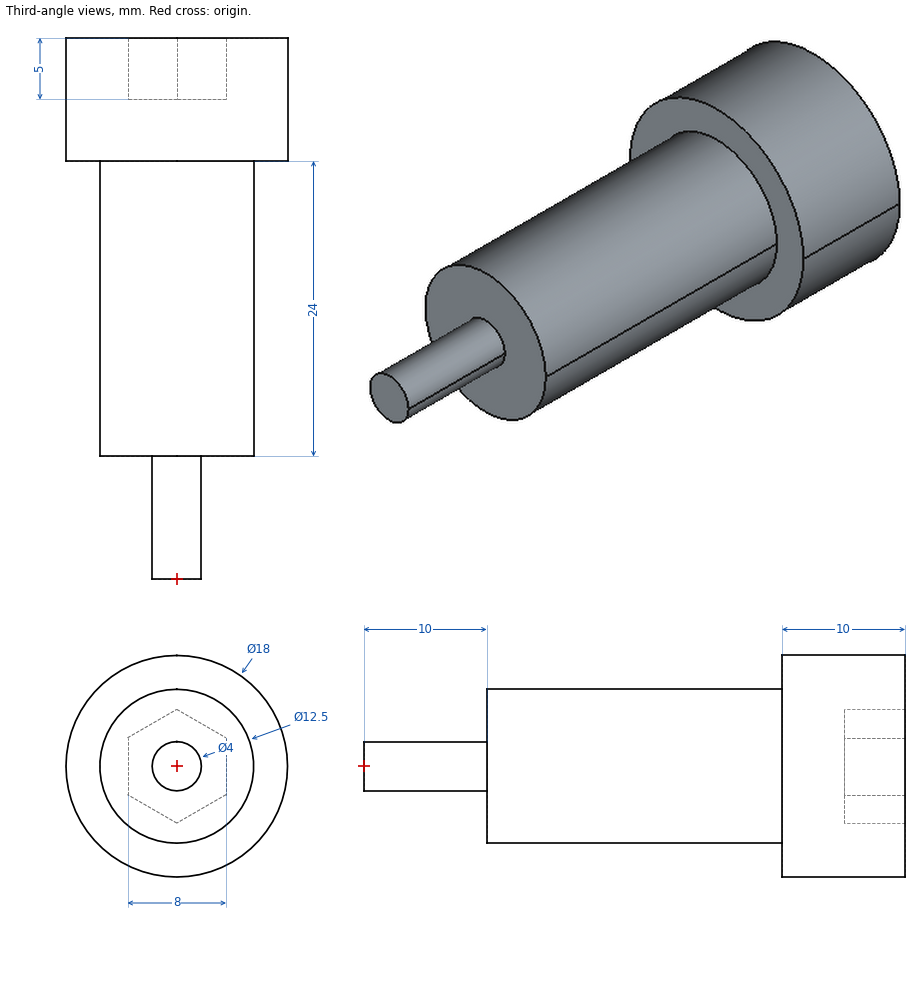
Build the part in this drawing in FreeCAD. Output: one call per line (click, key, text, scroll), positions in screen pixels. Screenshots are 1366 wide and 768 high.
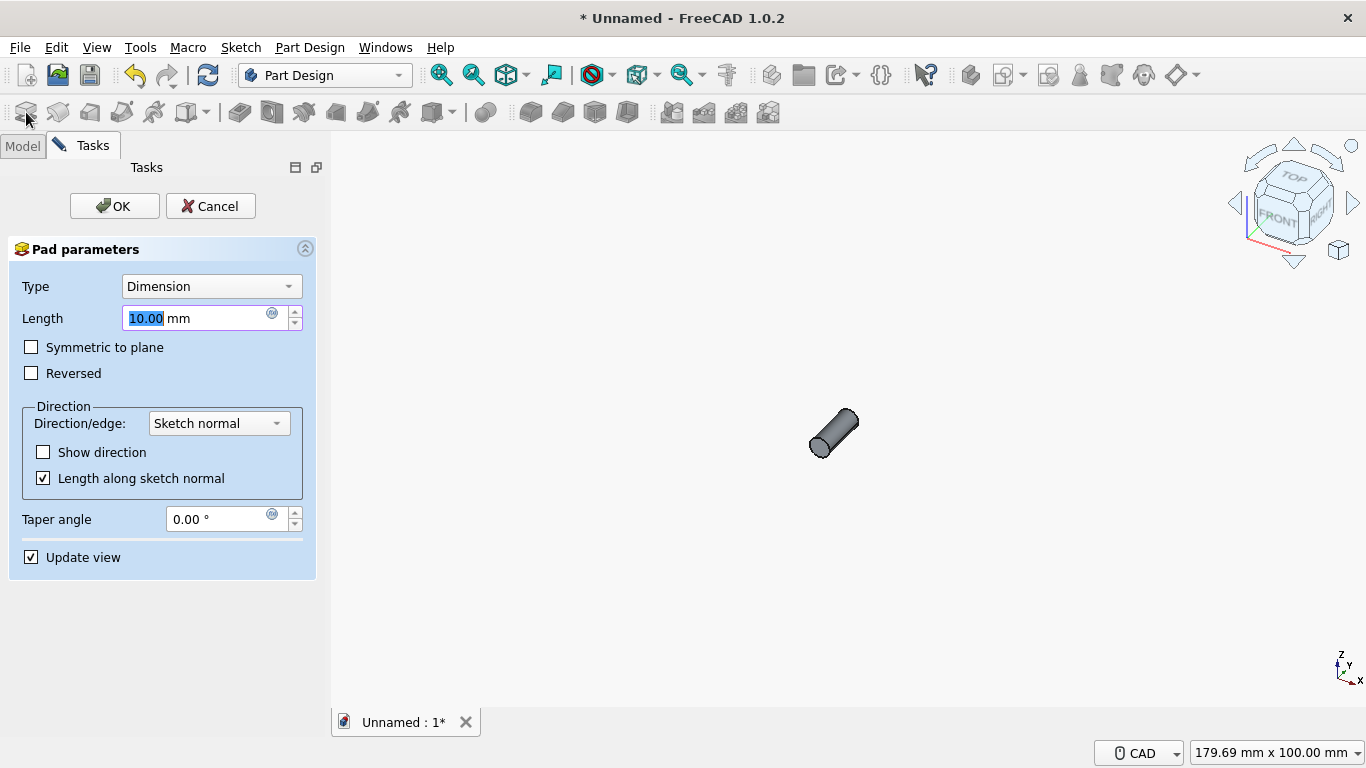
text(10)
key(Tab)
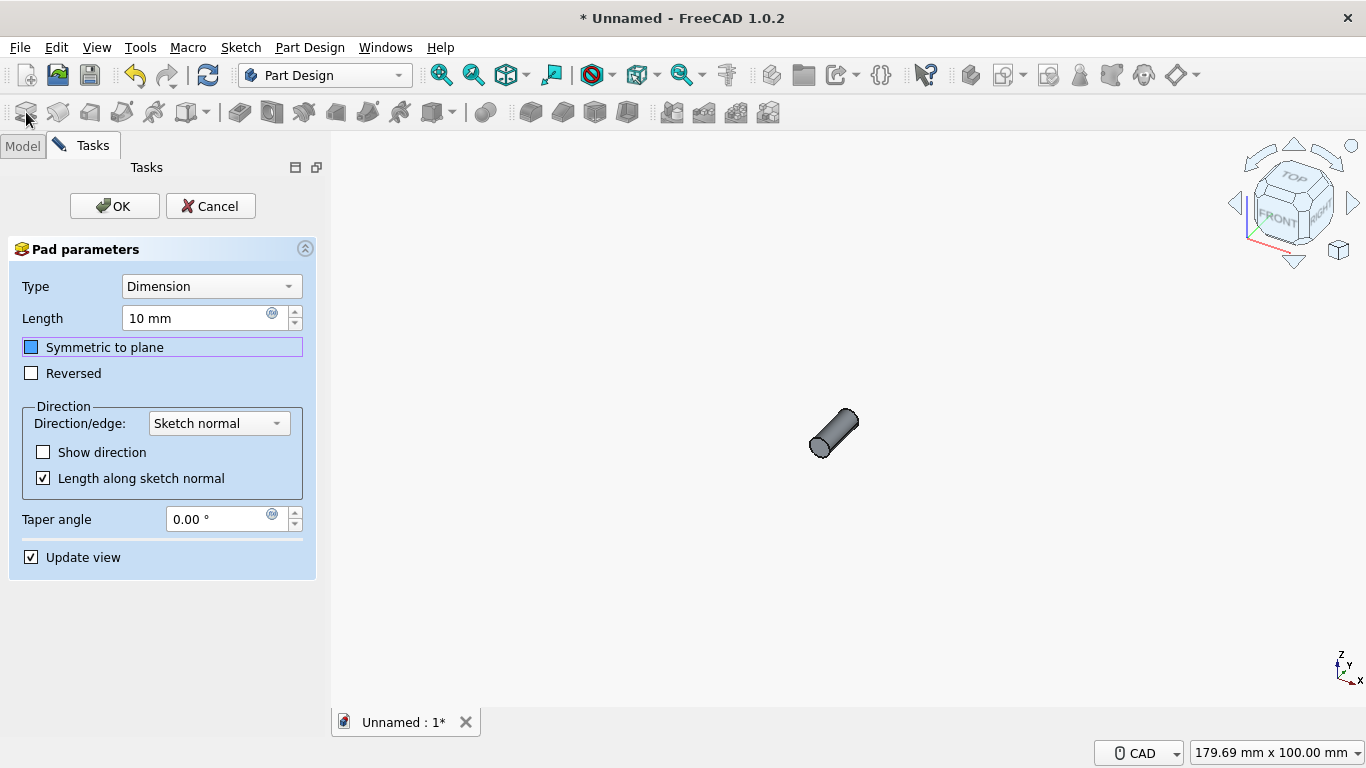
click(30, 373)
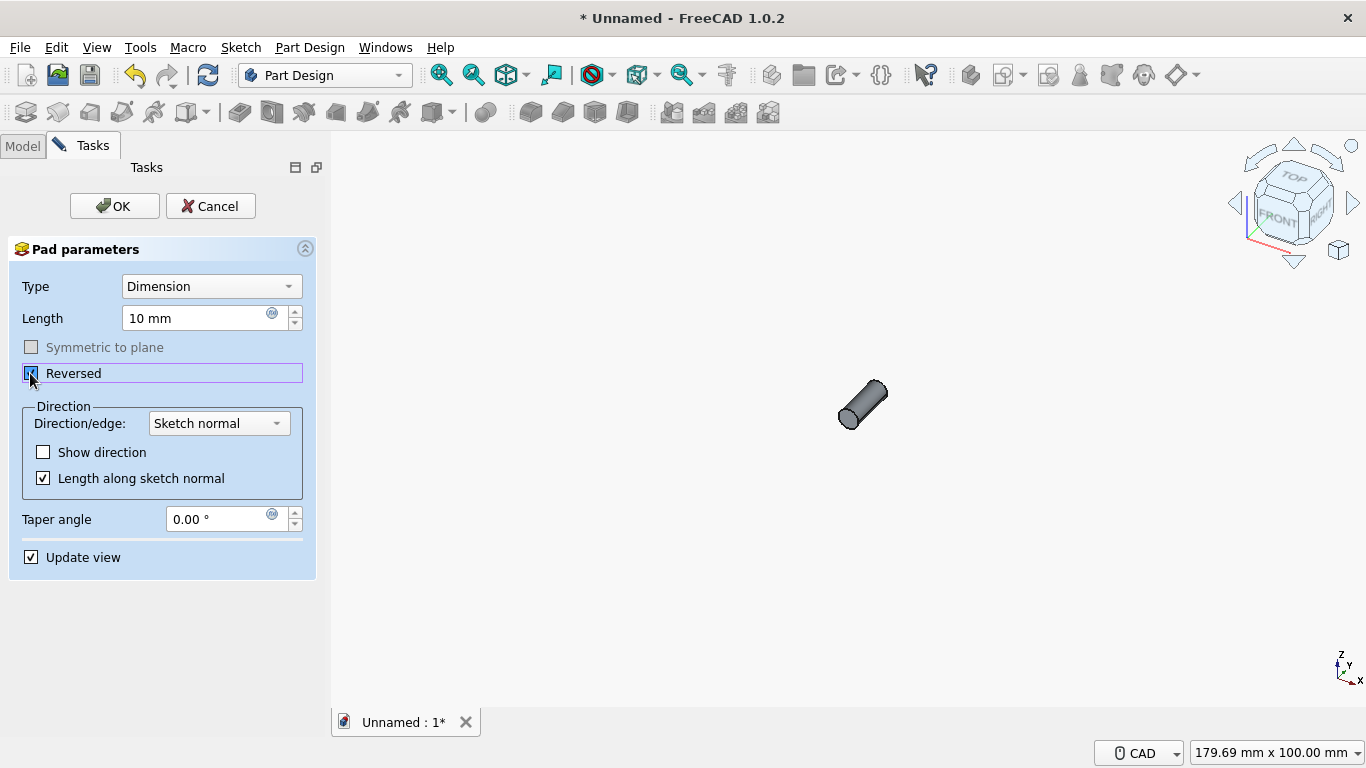
click(115, 206)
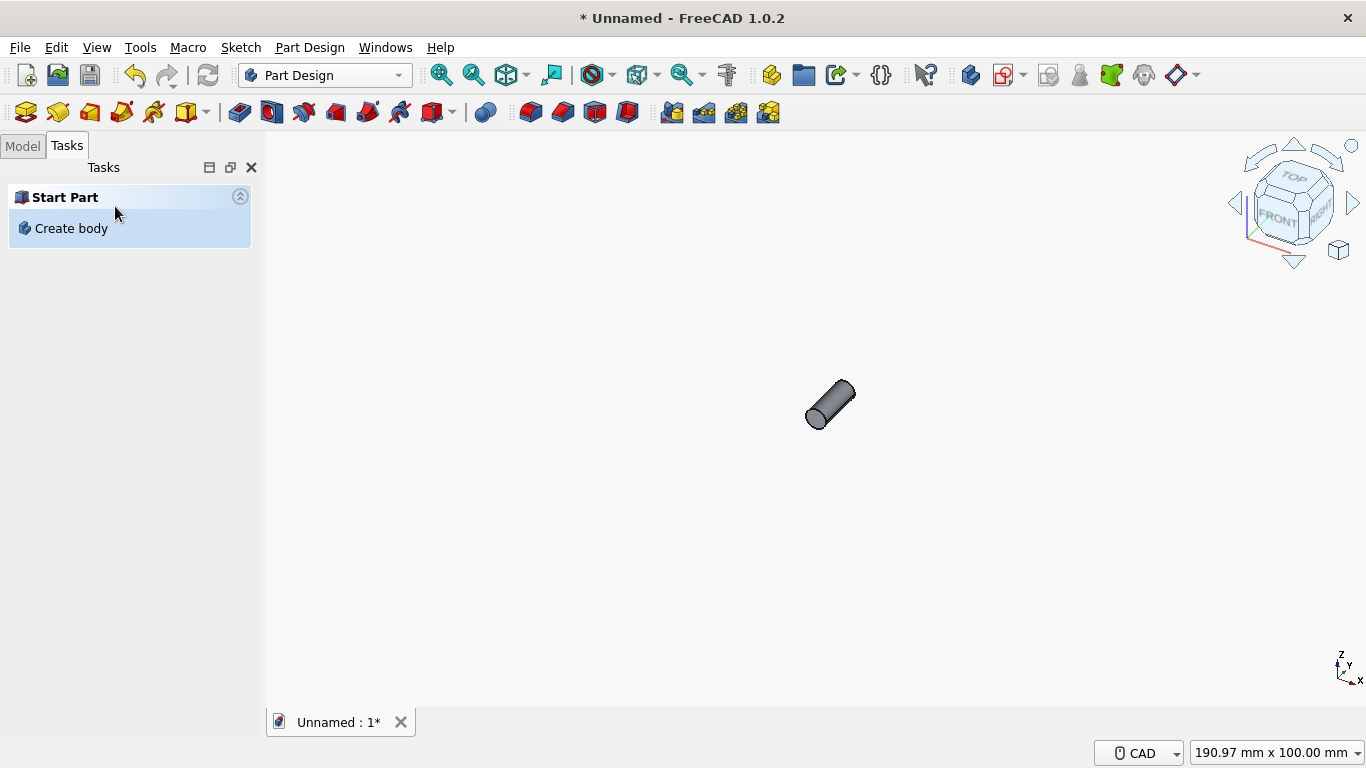
key(v)
key(f)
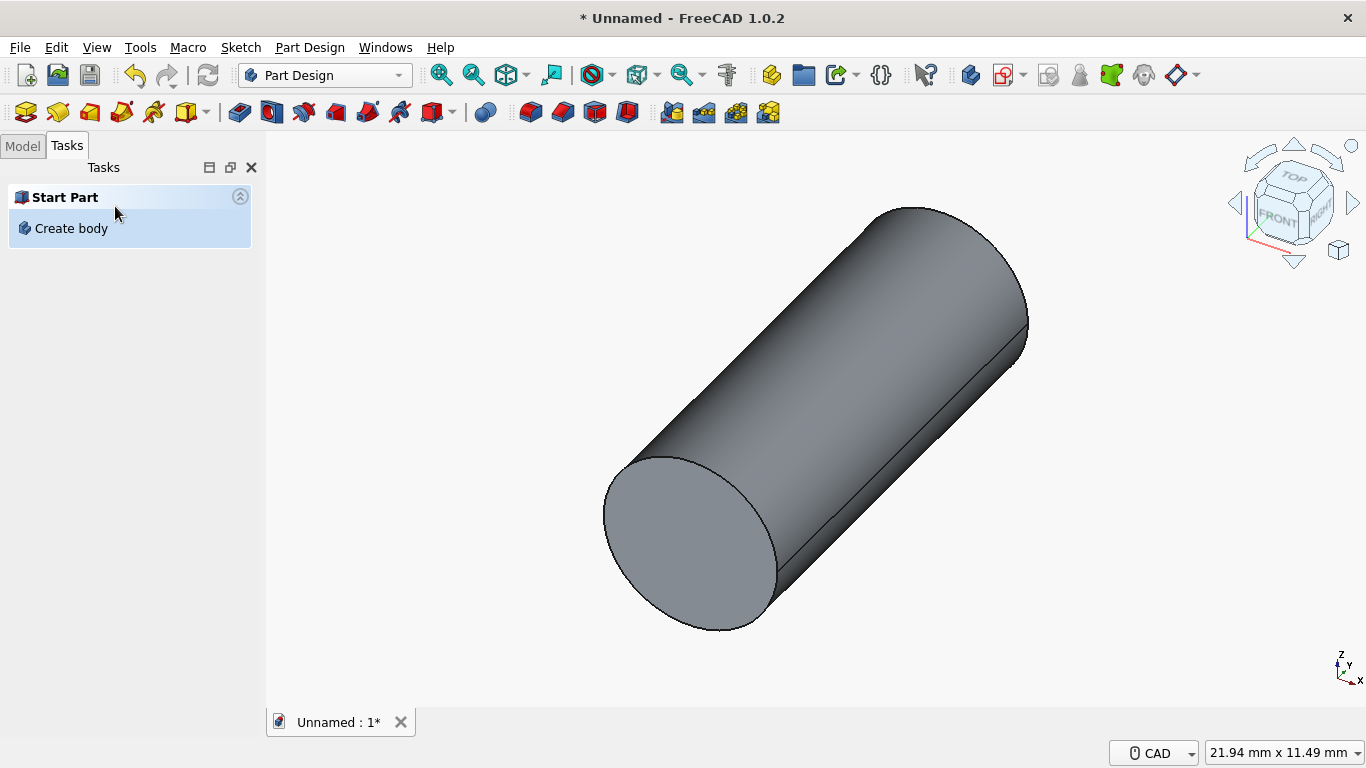
key(4)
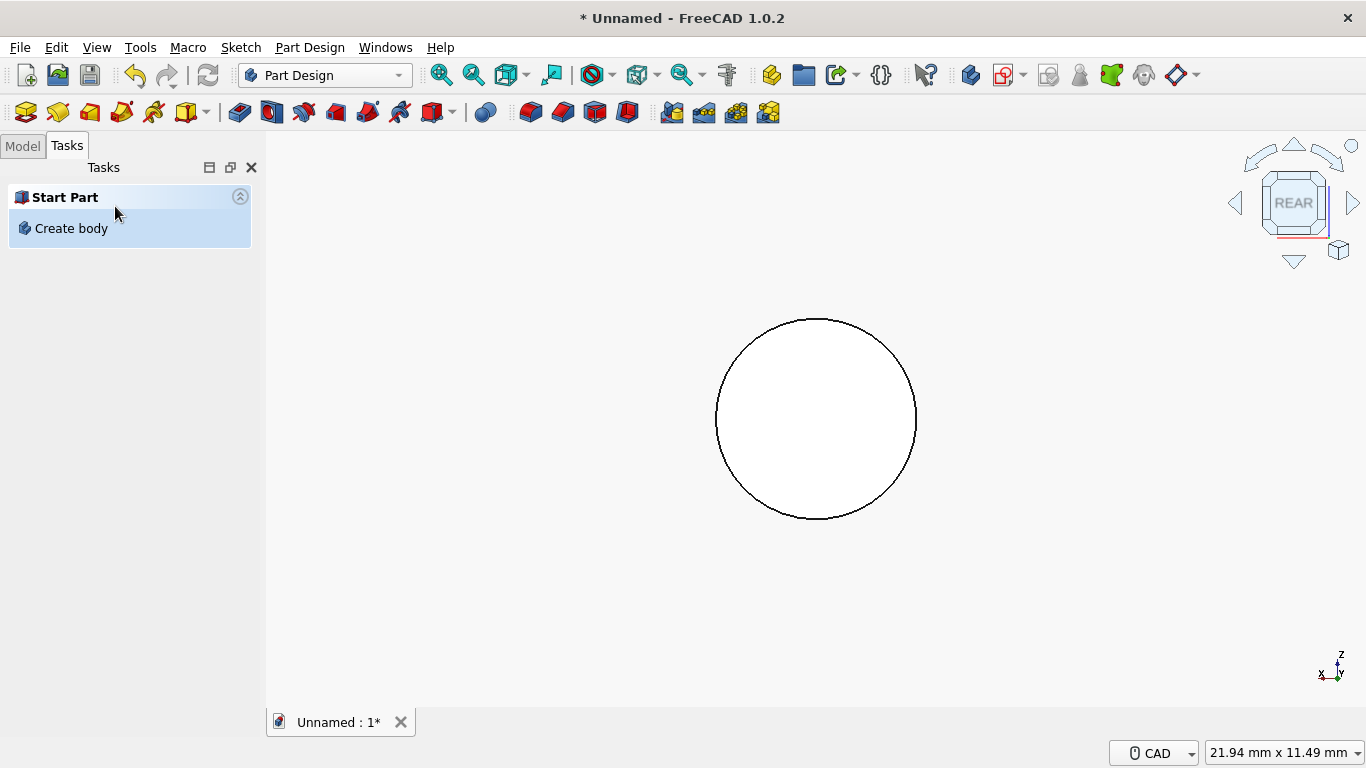
key(v)
key(f)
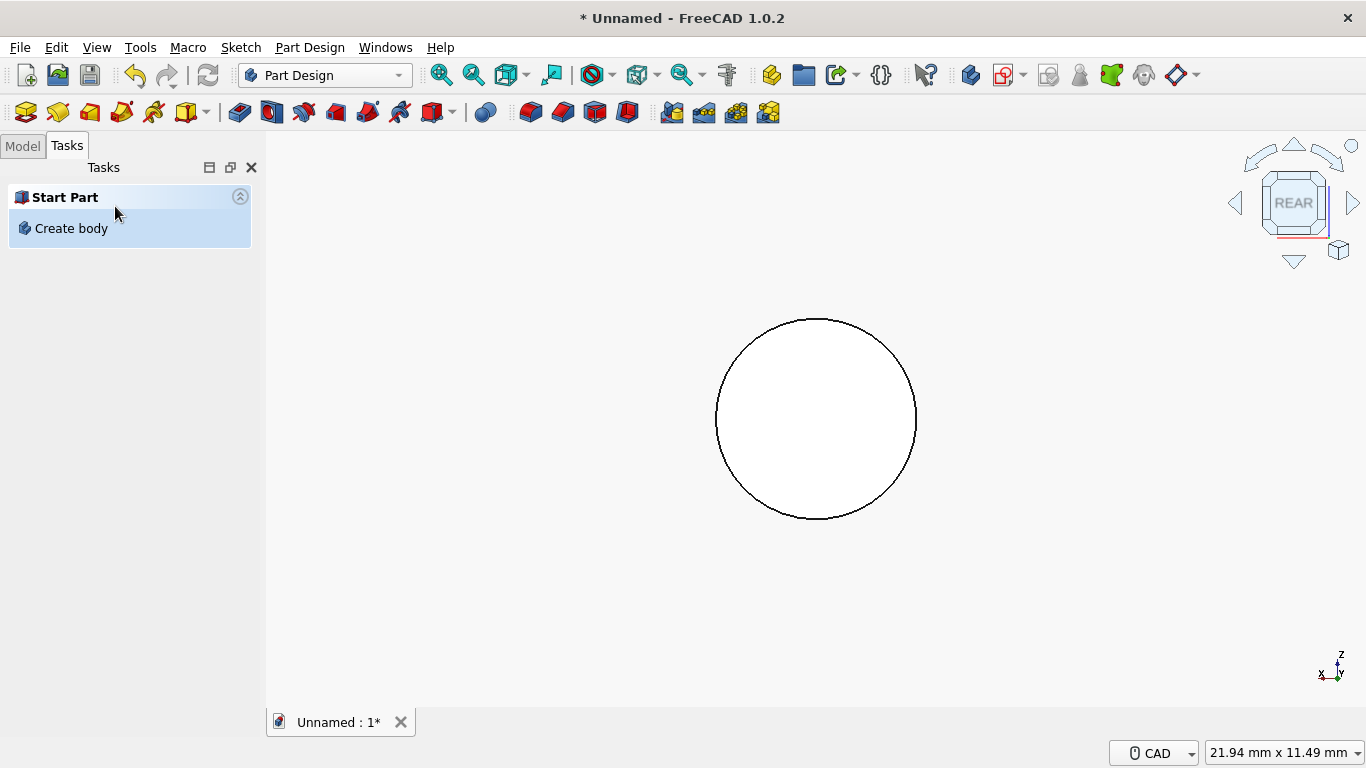
click(816, 418)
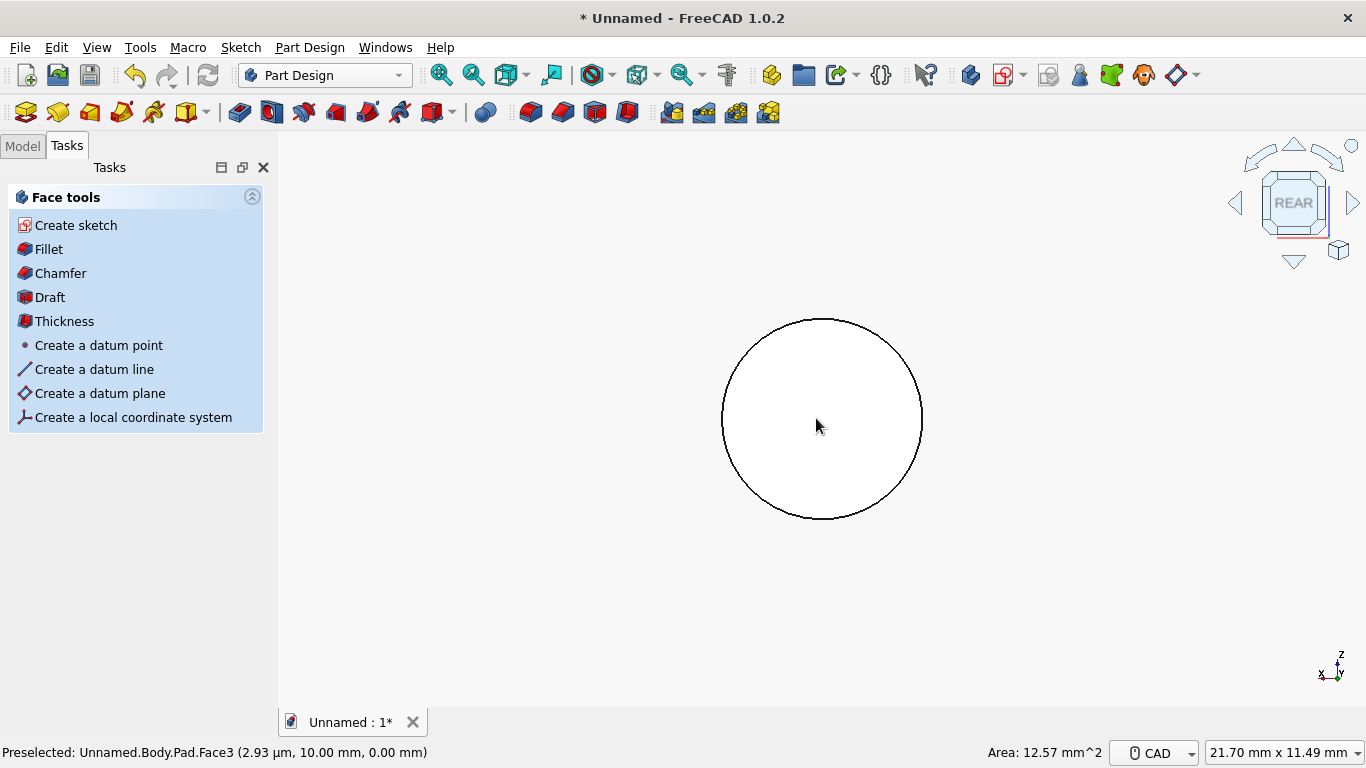
click(1004, 76)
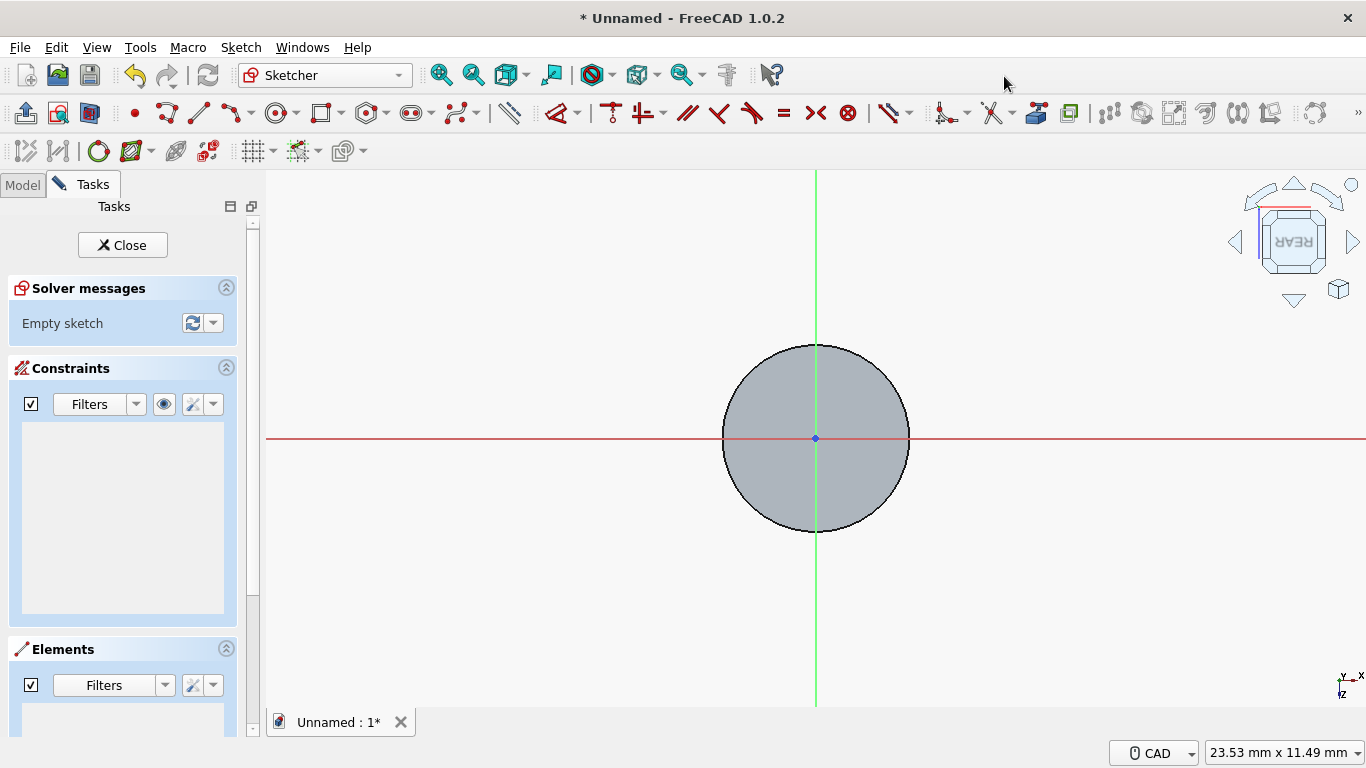
scroll(664, 439, down, 3)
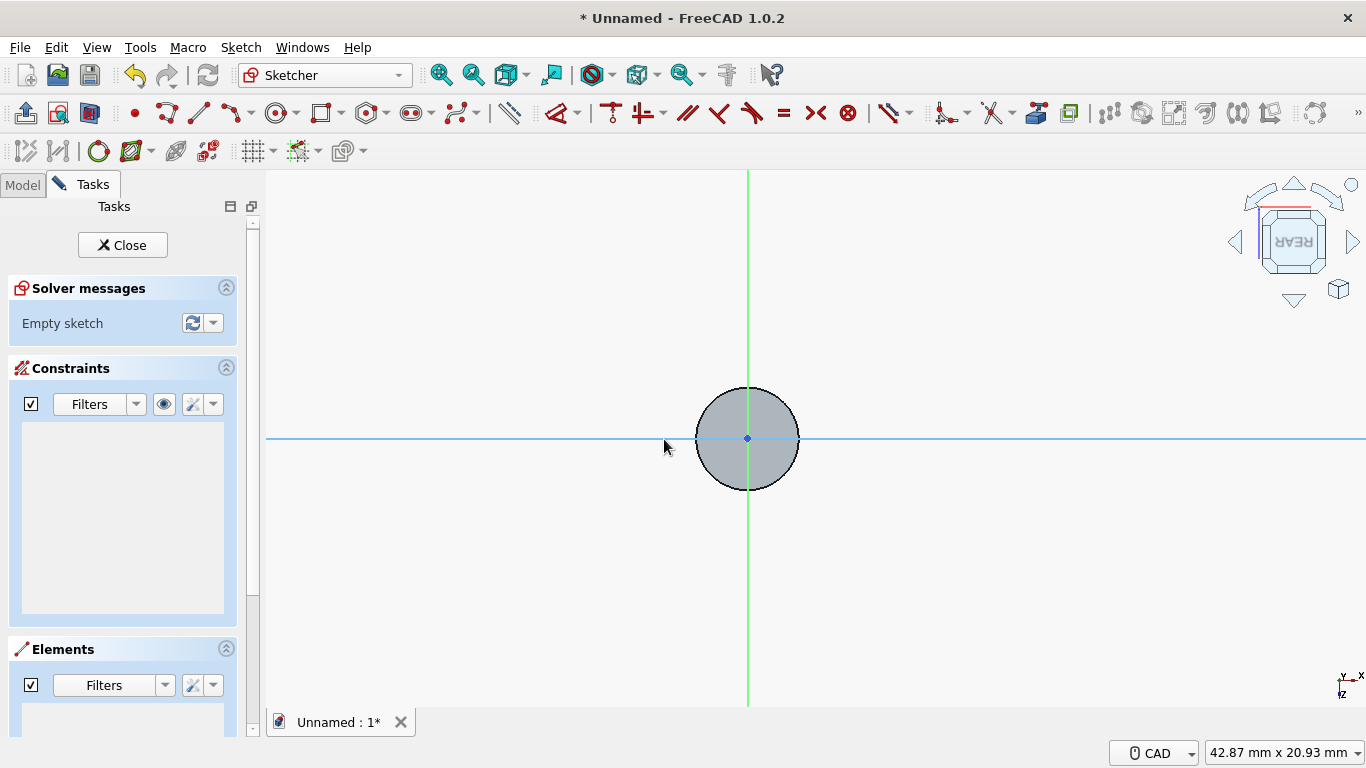
key(g)
key(c)